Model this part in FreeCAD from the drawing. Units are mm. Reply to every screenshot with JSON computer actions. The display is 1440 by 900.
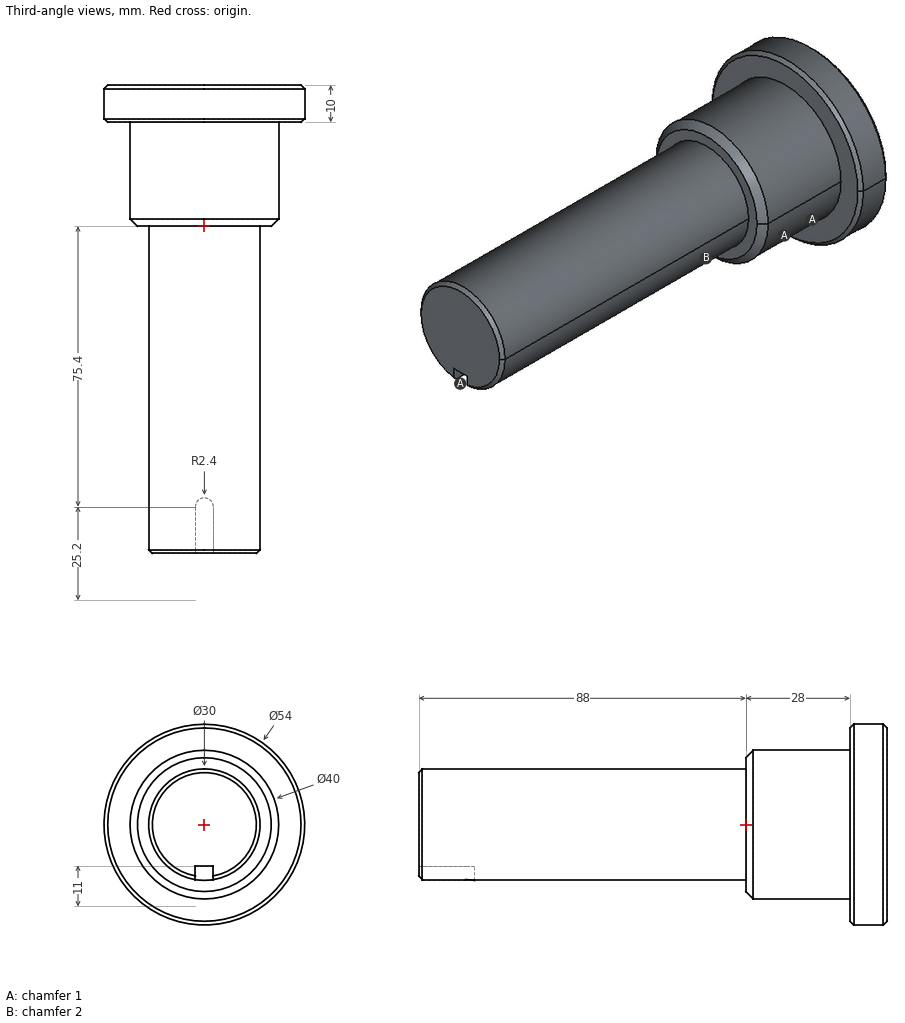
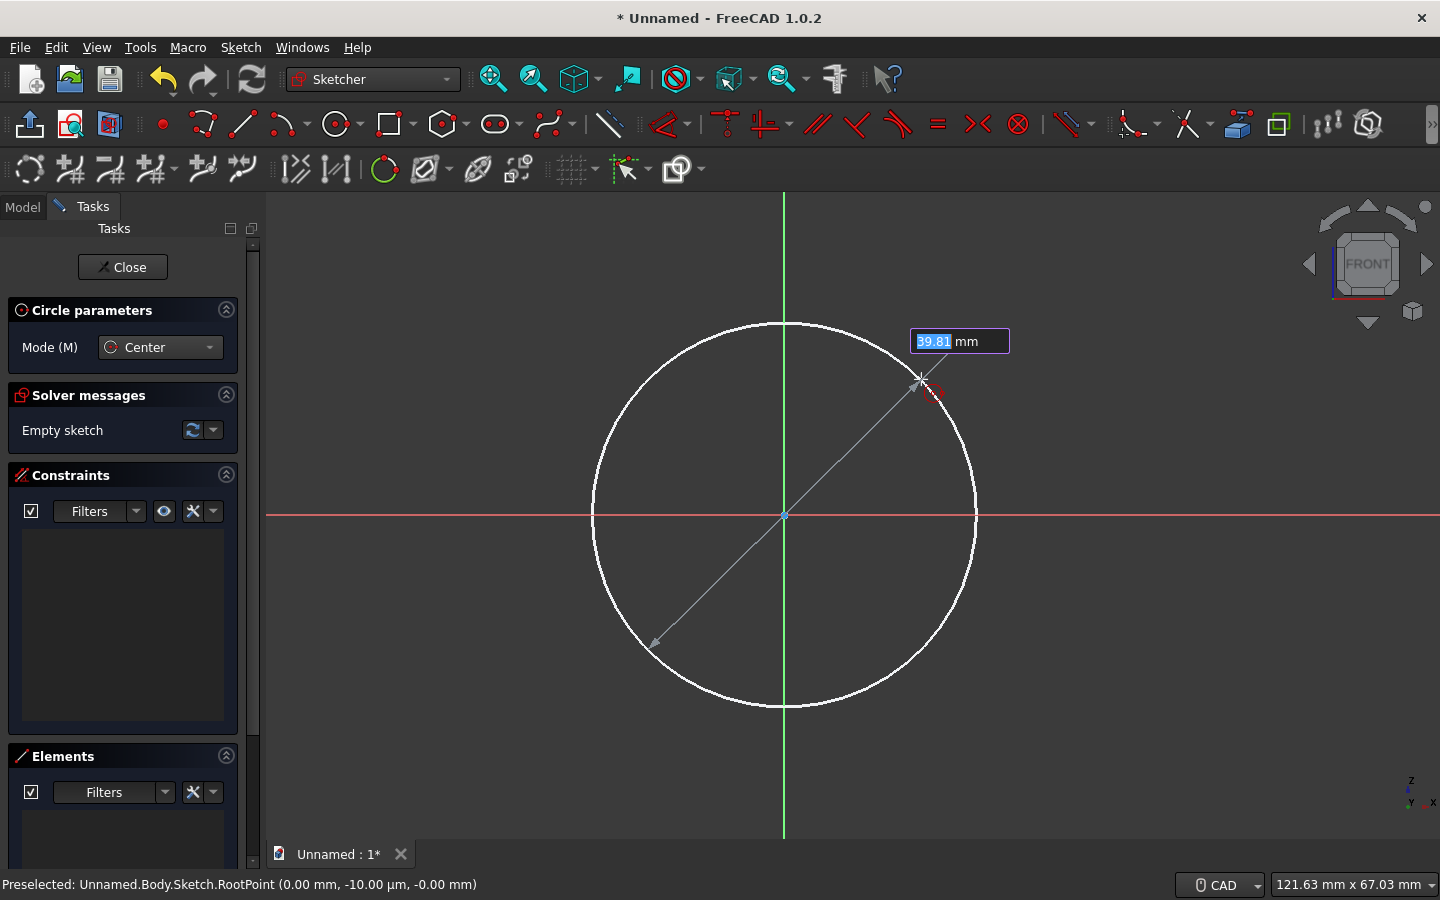
{"action": "type", "text": "40"}
{"action": "key", "text": "Return"}
{"action": "key", "text": "Escape"}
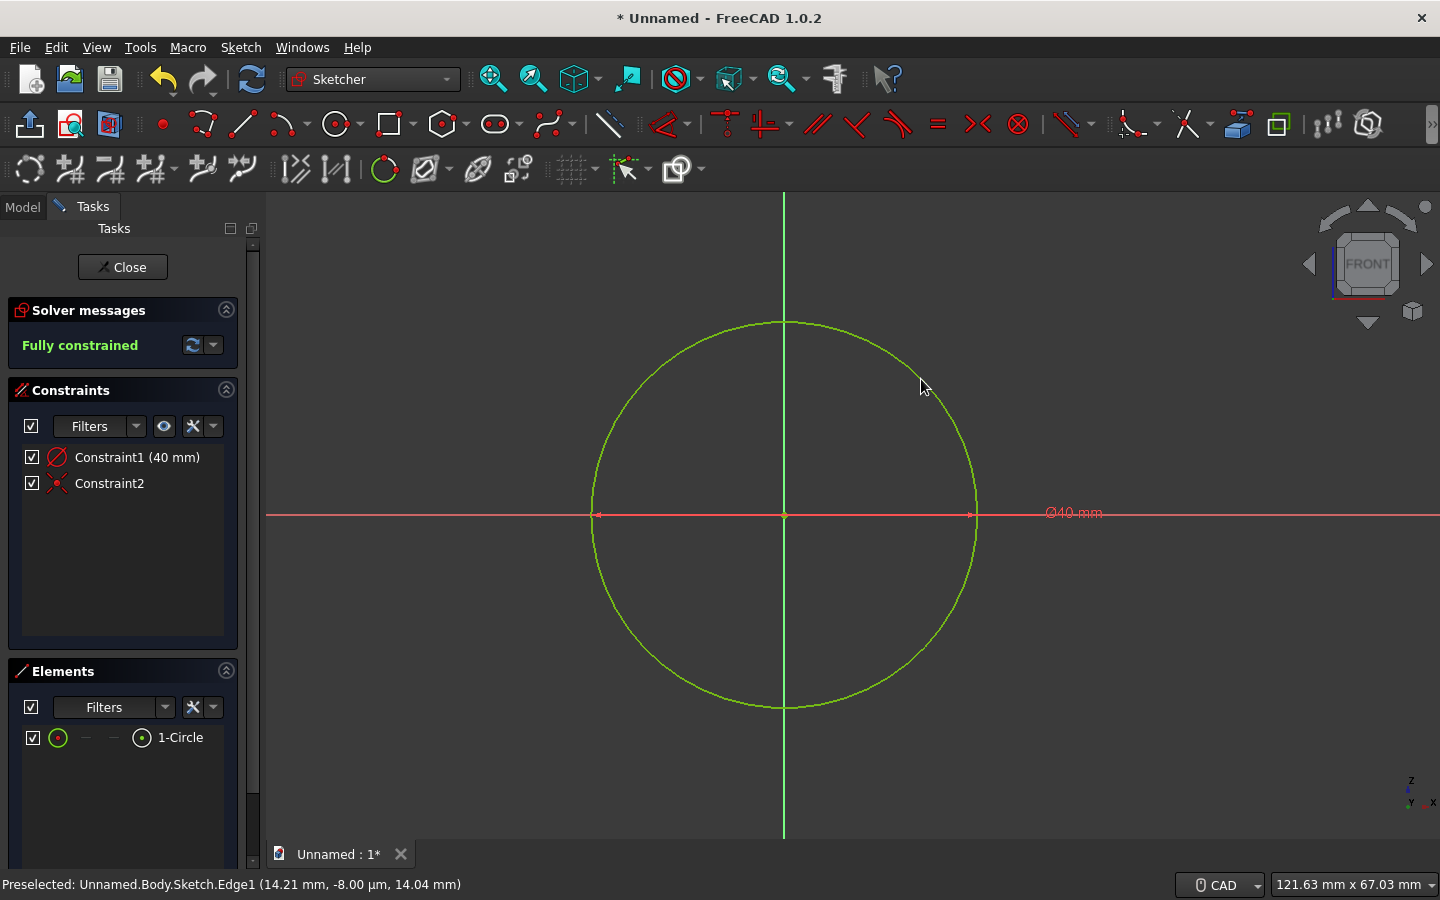
{"action": "left_click", "coordinate": [123, 267]}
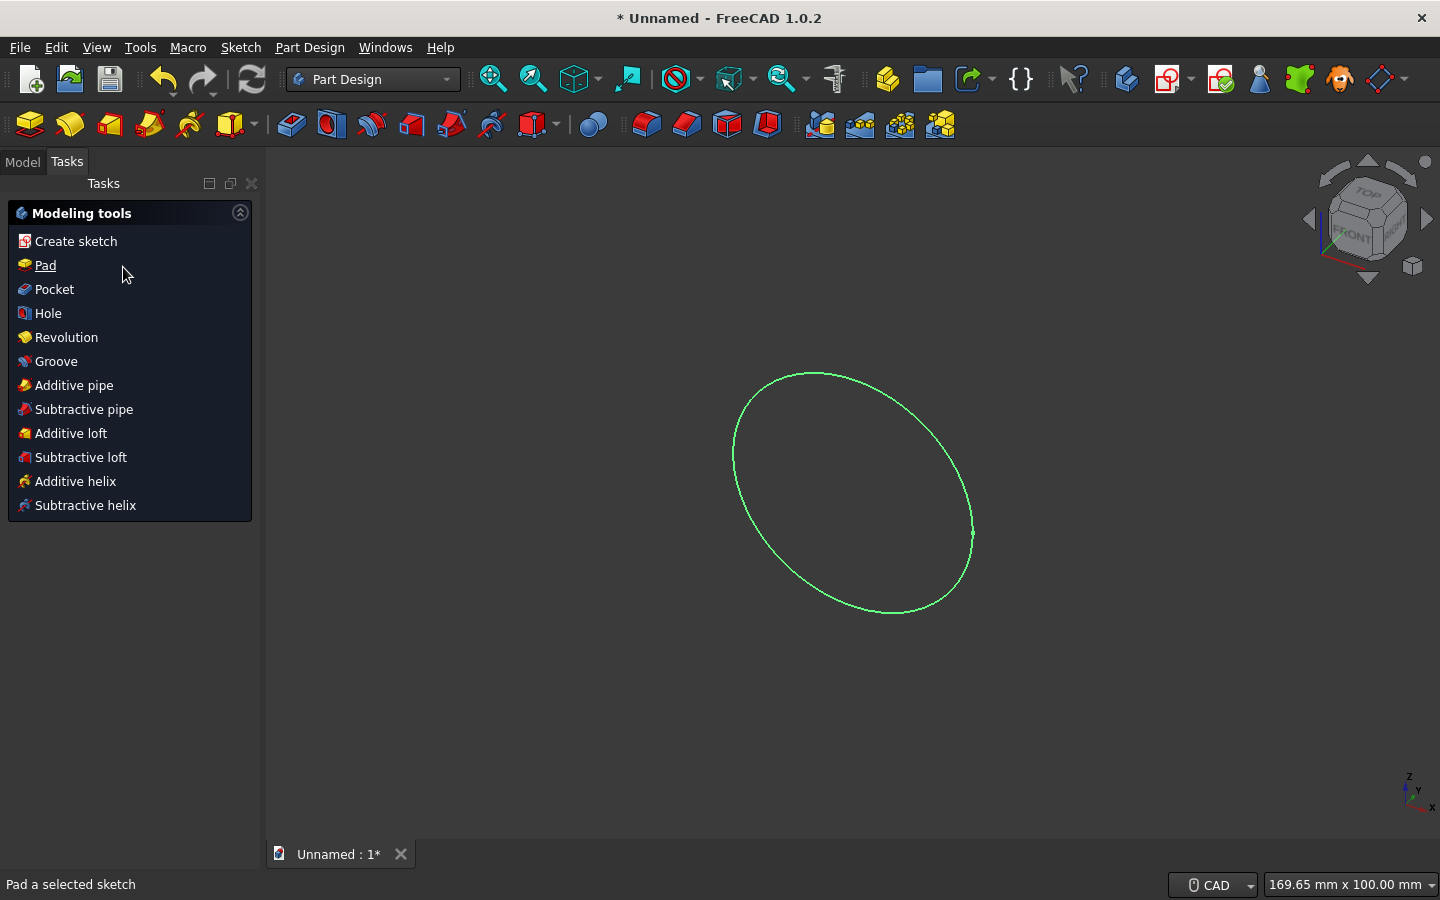
{"action": "left_click", "coordinate": [30, 124]}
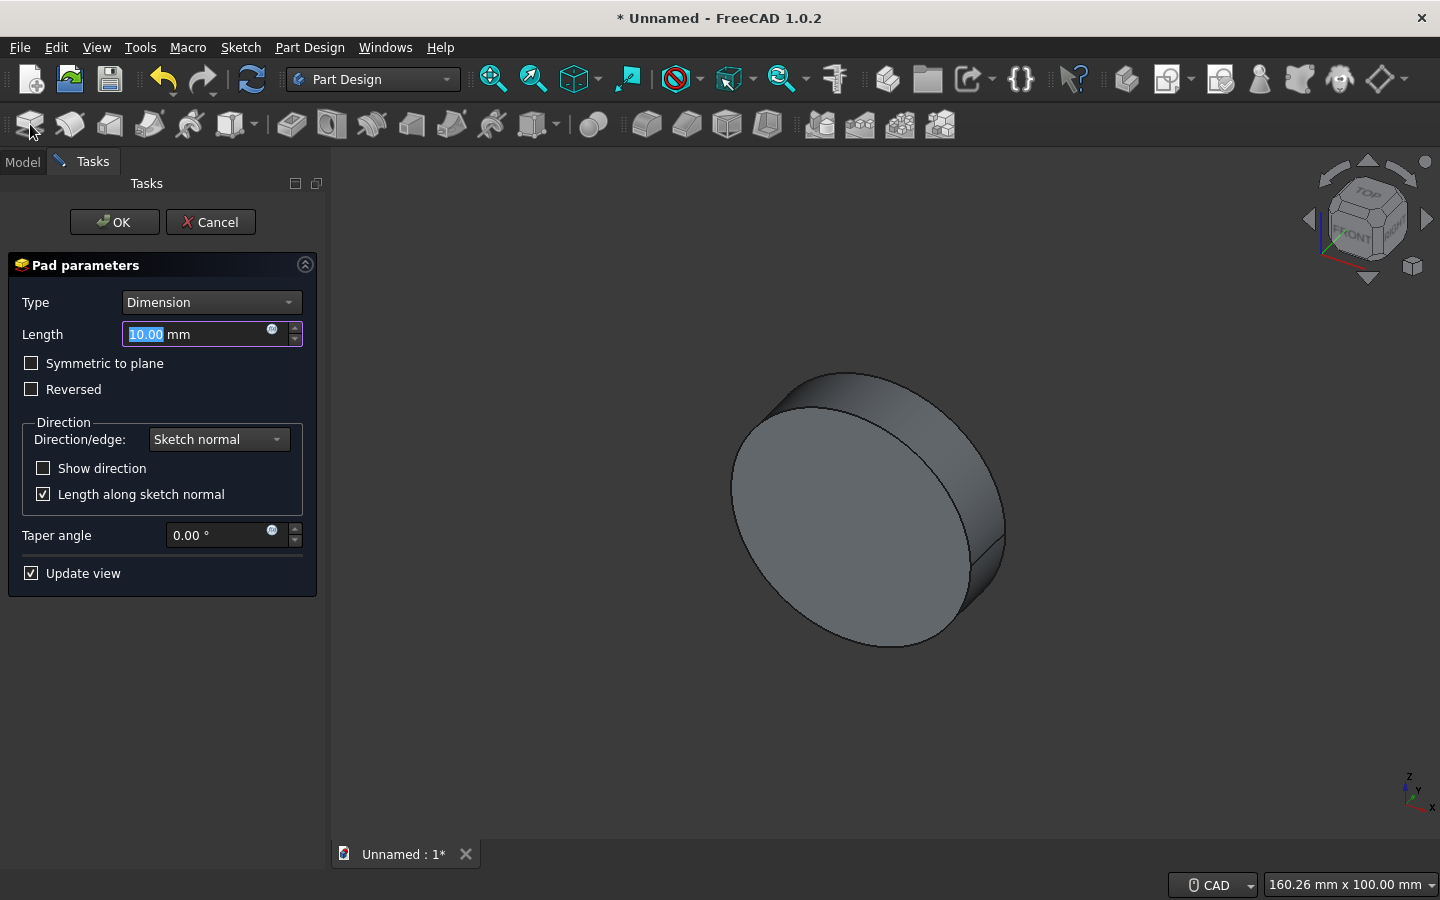
{"action": "type", "text": "28"}
{"action": "key", "text": "Tab"}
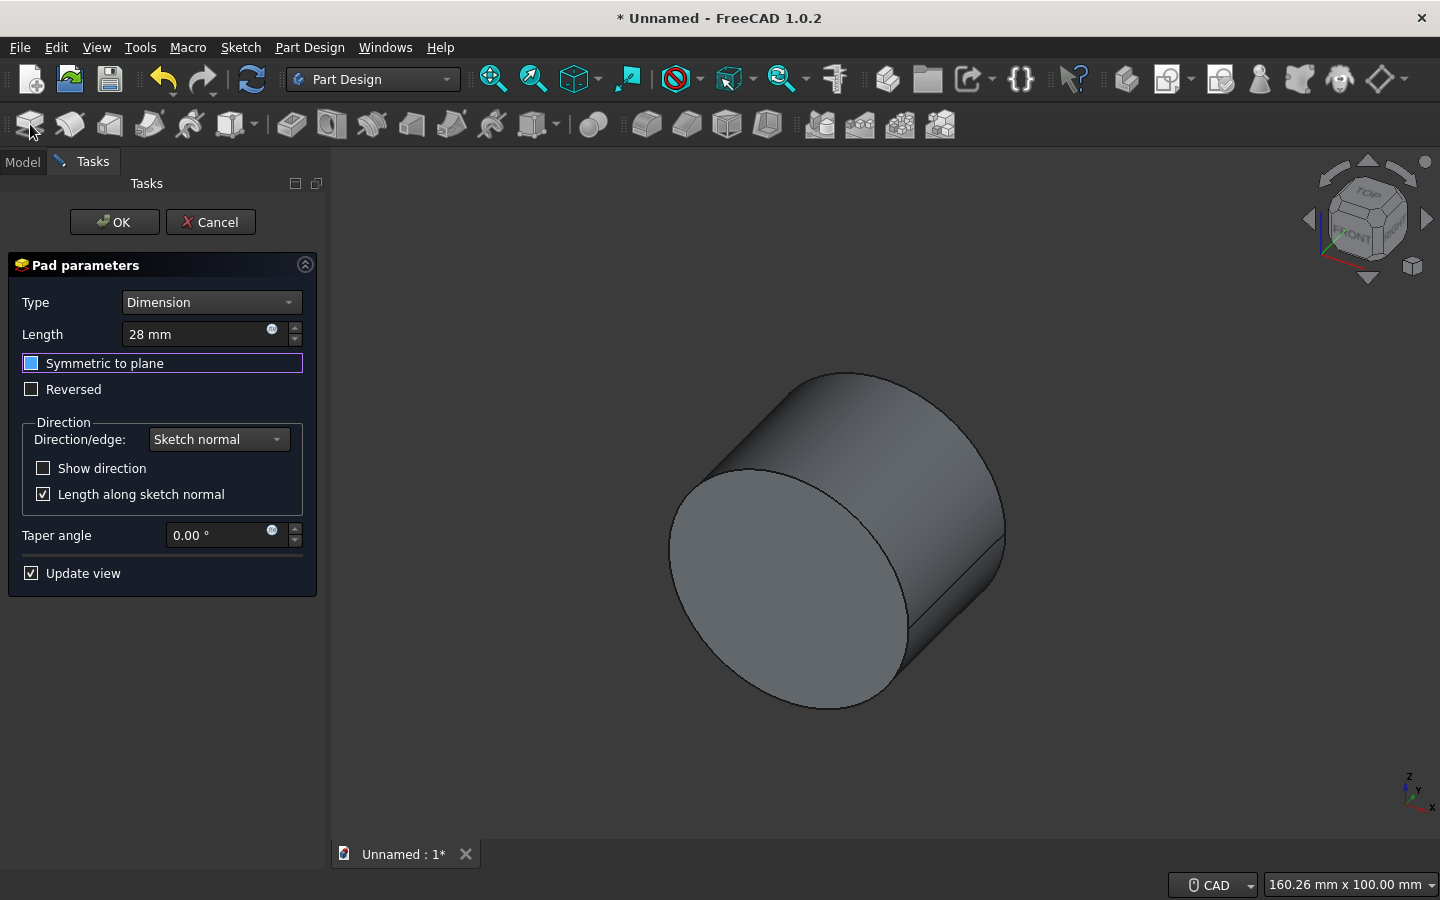
{"action": "left_click", "coordinate": [30, 389]}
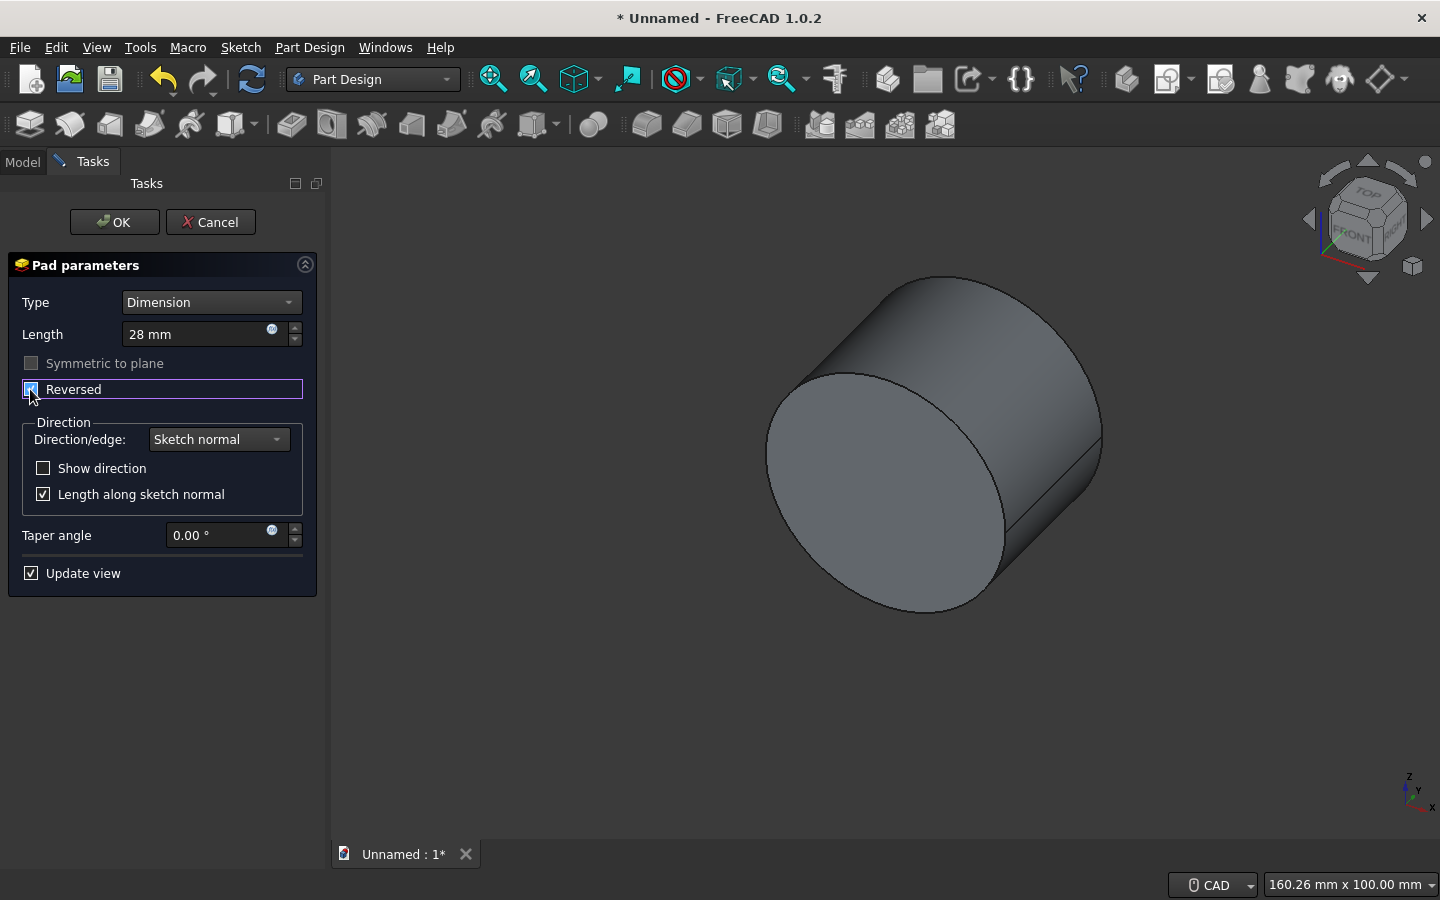
{"action": "left_click", "coordinate": [115, 222]}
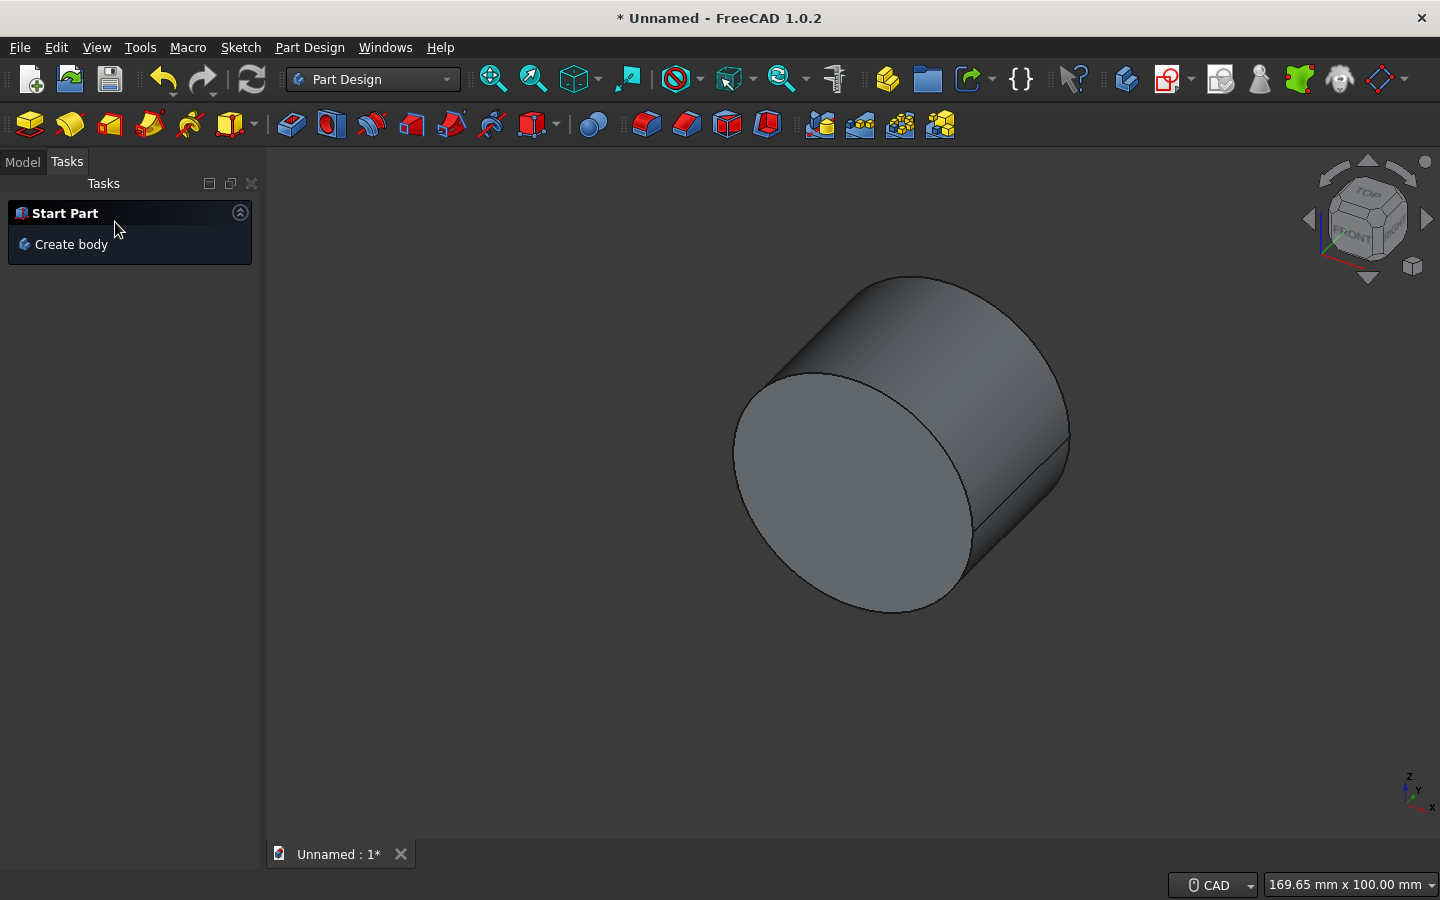
{"action": "key", "text": "4"}